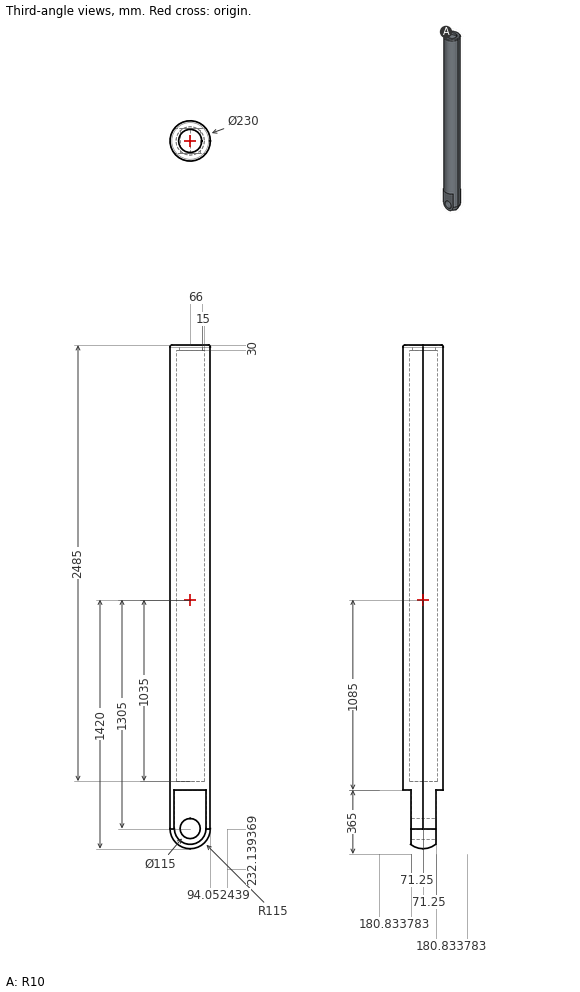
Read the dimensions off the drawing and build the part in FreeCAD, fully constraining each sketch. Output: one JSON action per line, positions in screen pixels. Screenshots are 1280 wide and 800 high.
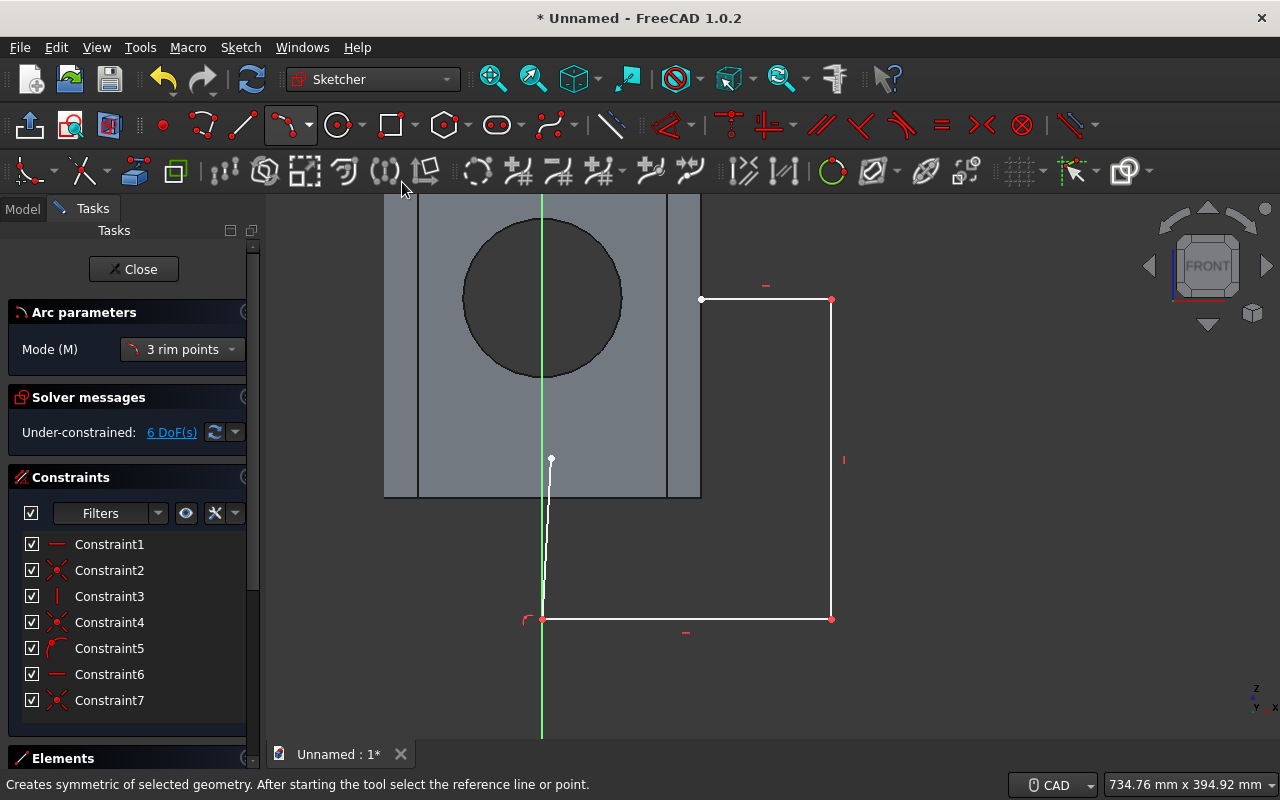
{"action": "left_click", "coordinate": [551, 458]}
{"action": "left_click", "coordinate": [701, 299]}
{"action": "left_click", "coordinate": [655, 410]}
{"action": "key", "text": "Escape"}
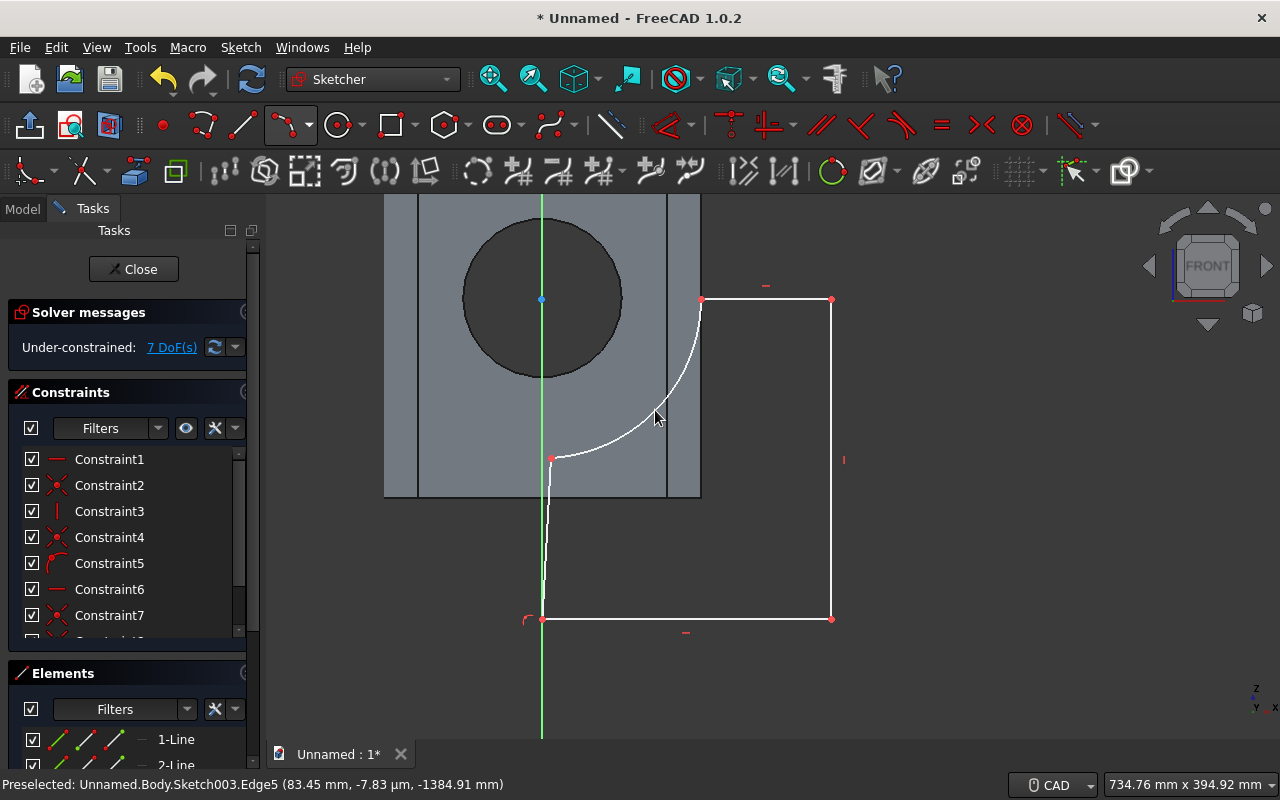
{"action": "left_click", "coordinate": [545, 571]}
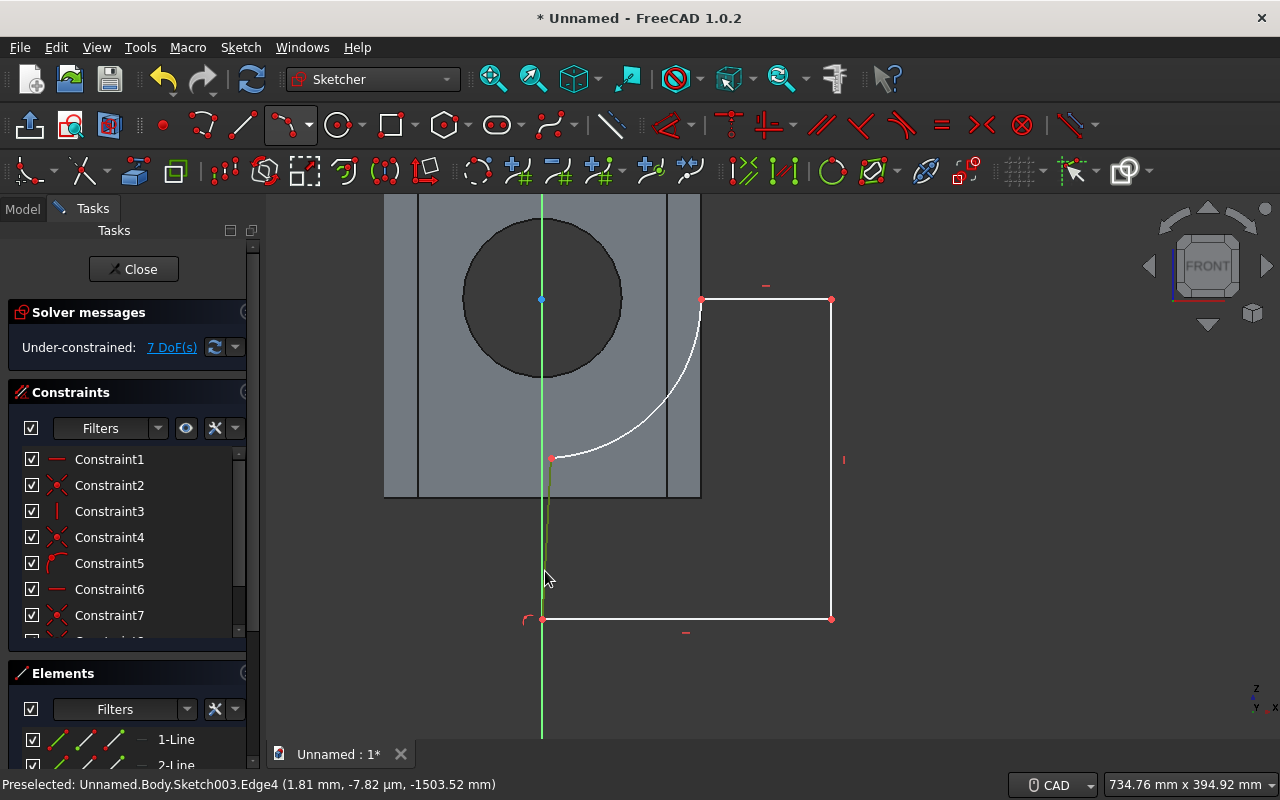
{"action": "left_click", "coordinate": [796, 126]}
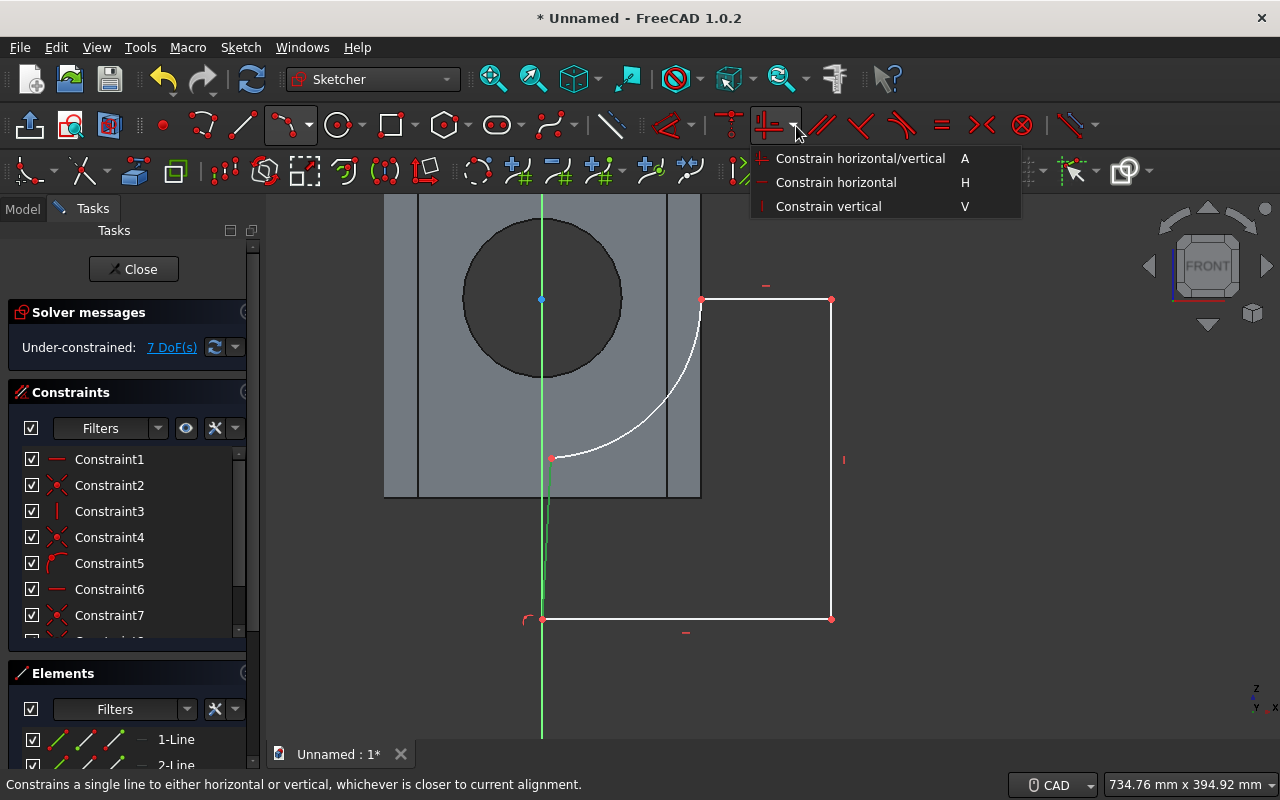
{"action": "left_click", "coordinate": [886, 206]}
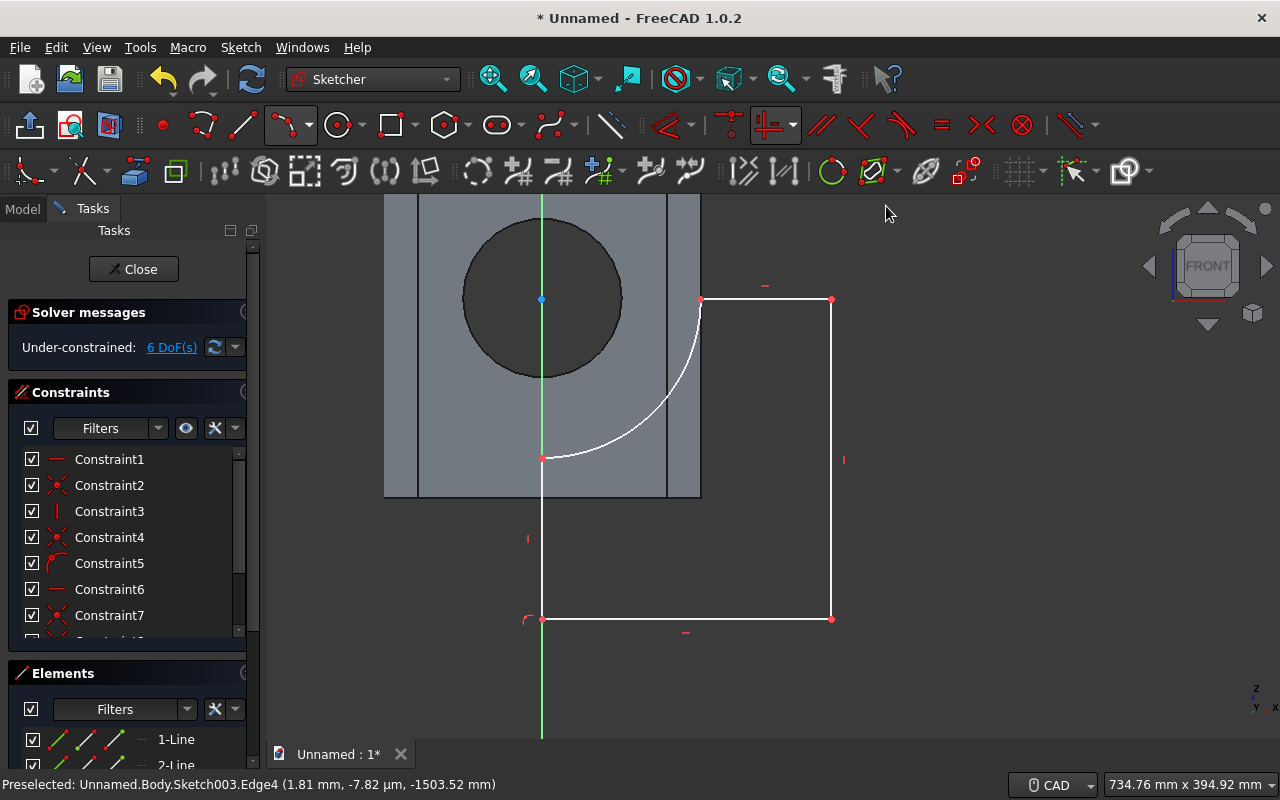
{"action": "left_click", "coordinate": [542, 299]}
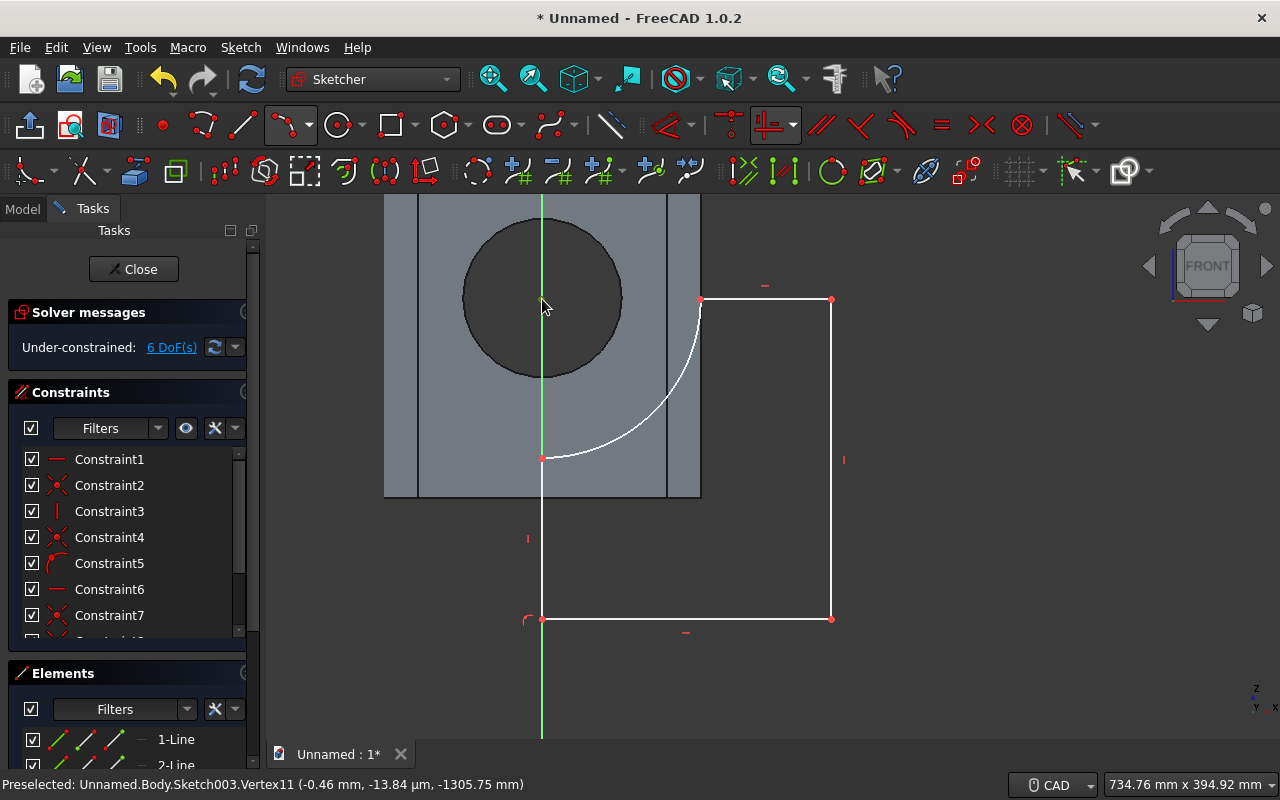
{"action": "left_click", "coordinate": [542, 676]}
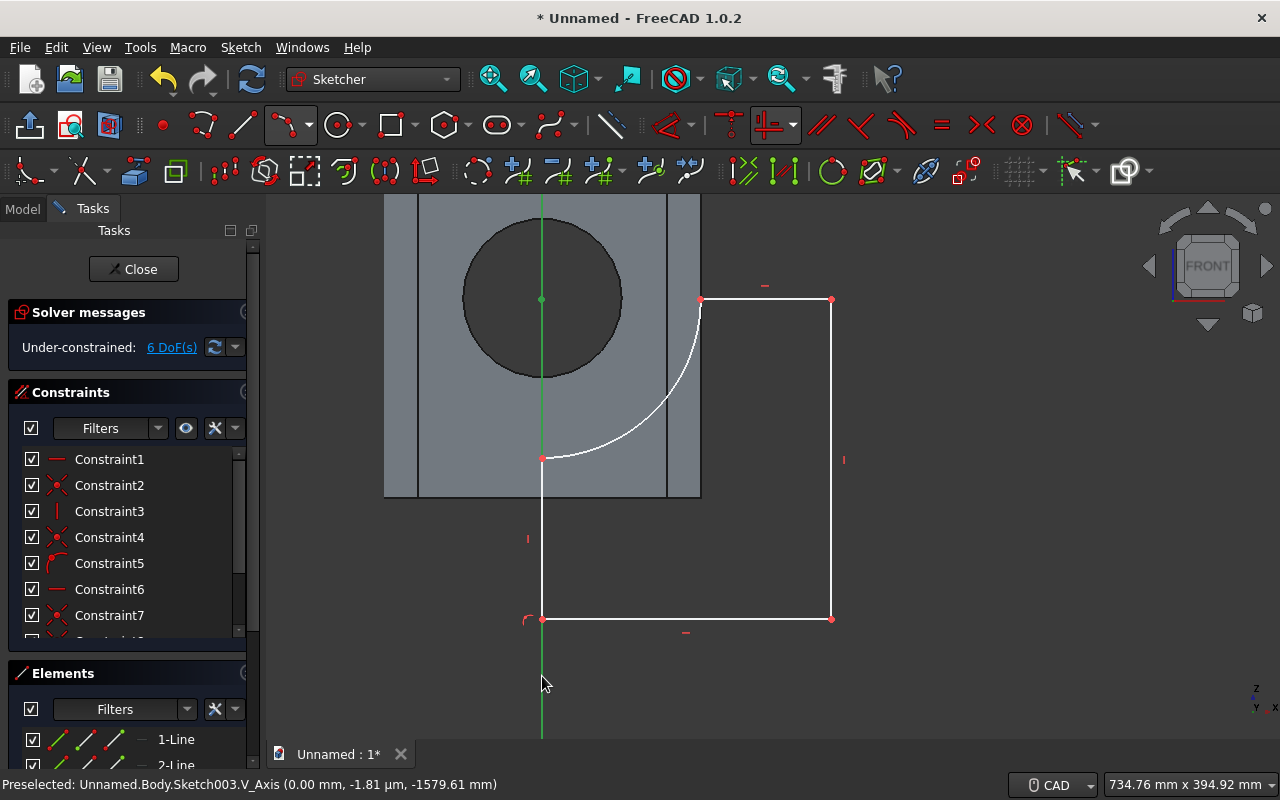
{"action": "key", "text": "c"}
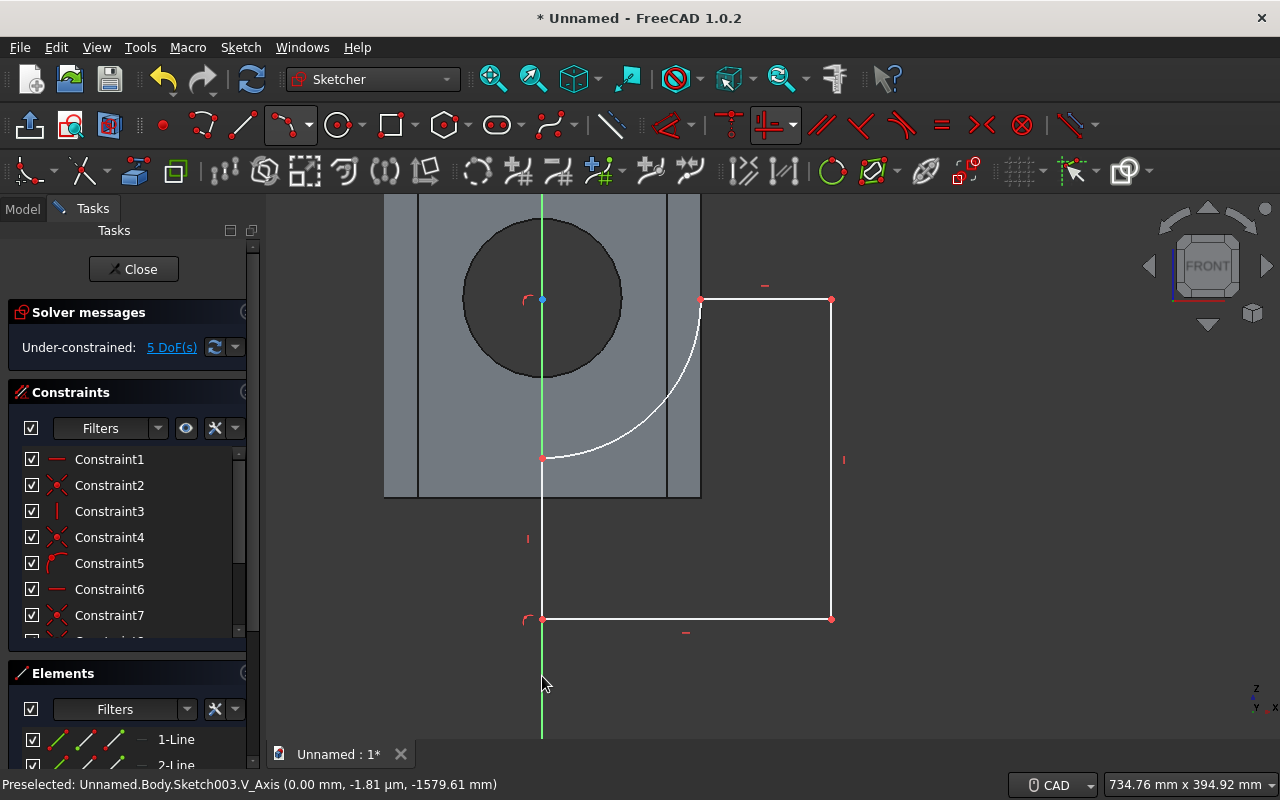
{"action": "key", "text": "d"}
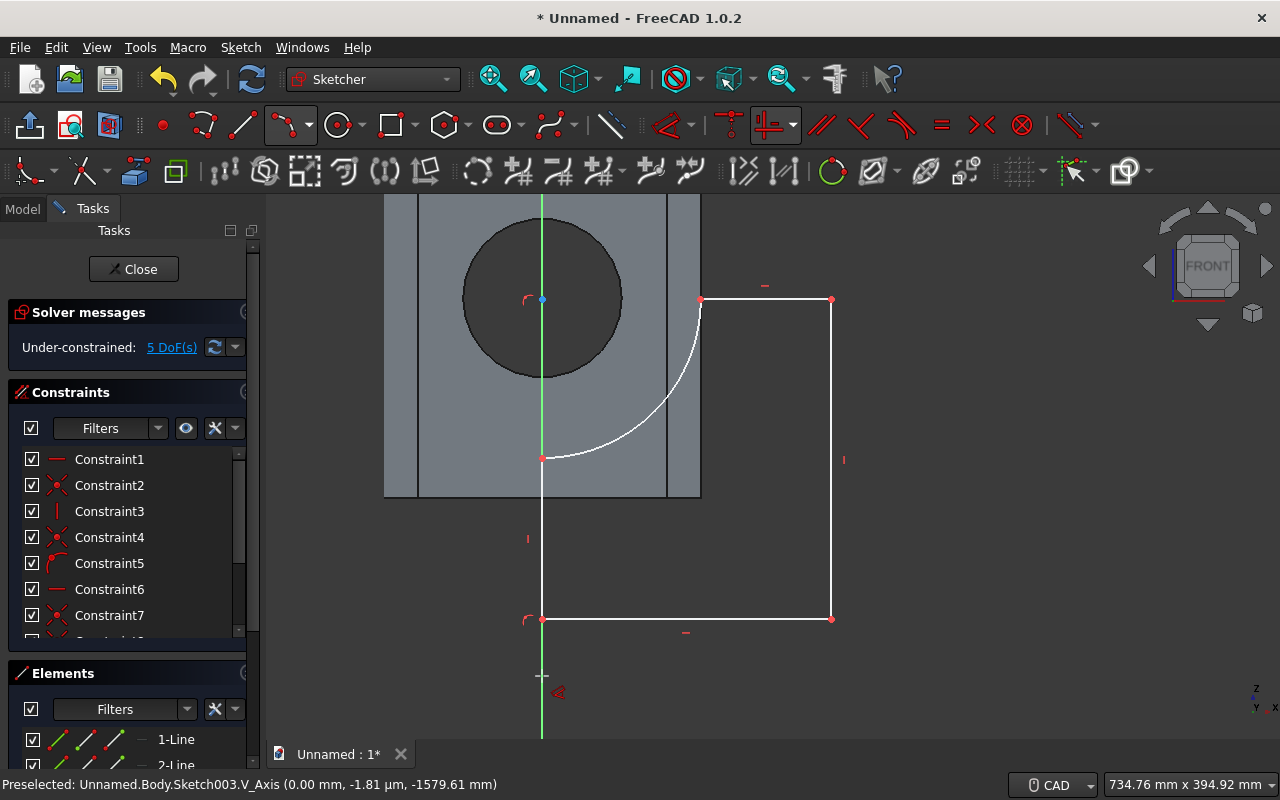
{"action": "left_click", "coordinate": [614, 441]}
{"action": "left_click", "coordinate": [628, 470]}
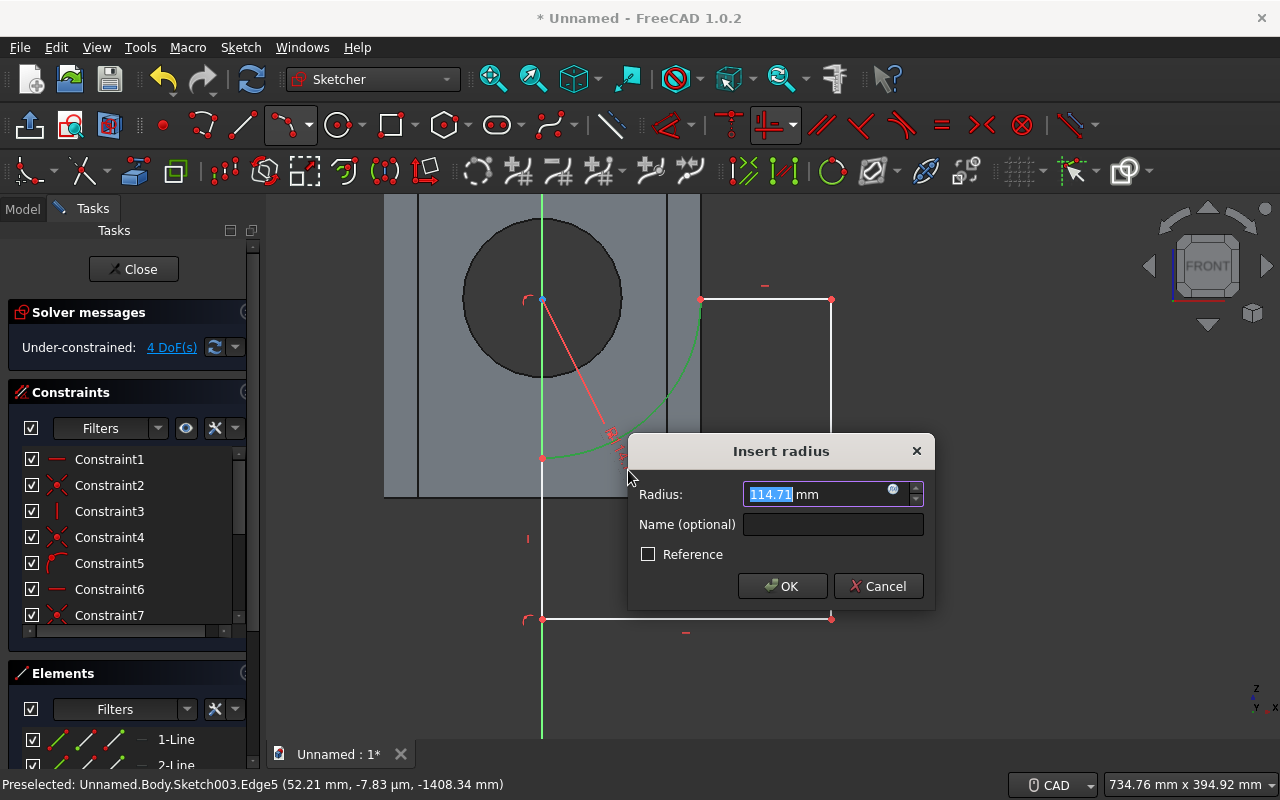
{"action": "type", "text": "115"}
{"action": "key", "text": "Return"}